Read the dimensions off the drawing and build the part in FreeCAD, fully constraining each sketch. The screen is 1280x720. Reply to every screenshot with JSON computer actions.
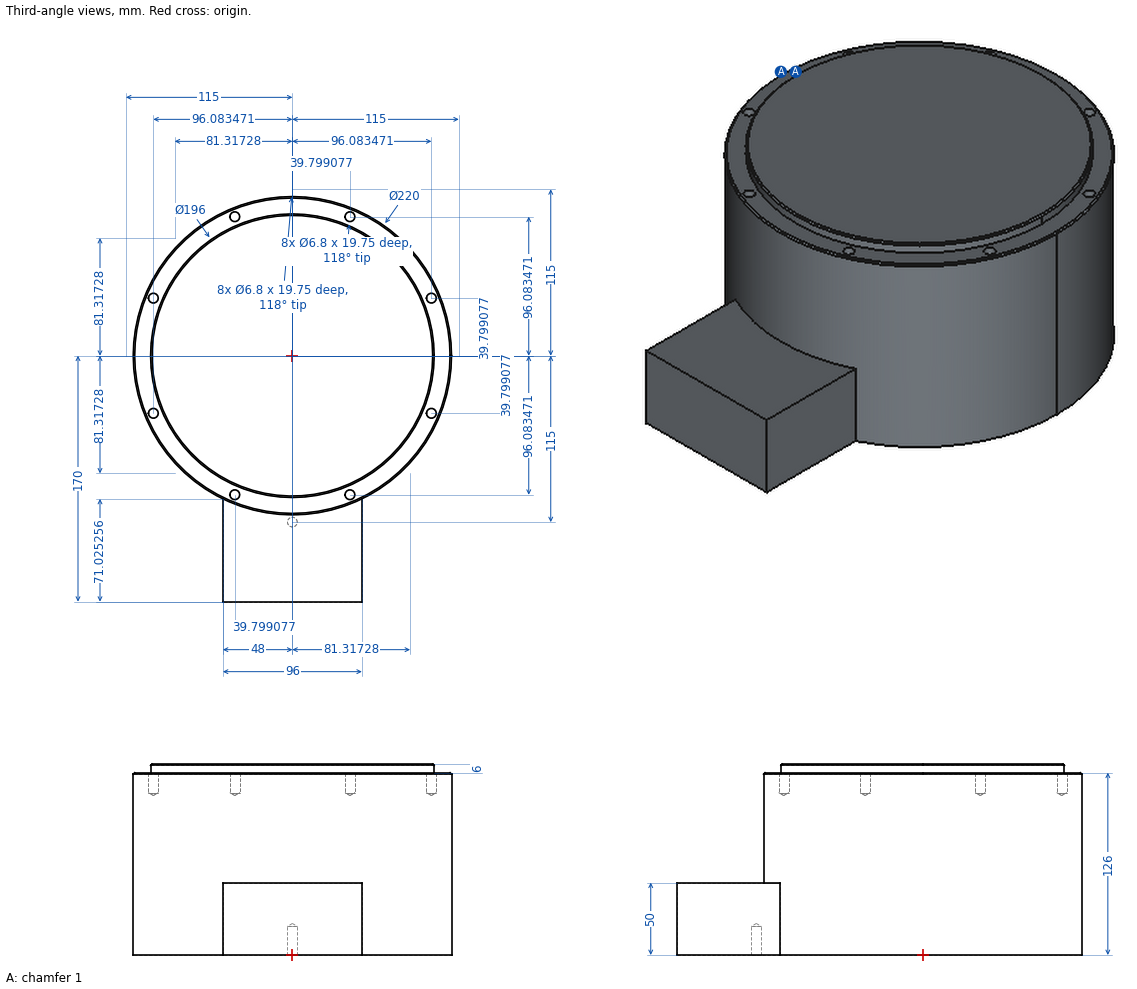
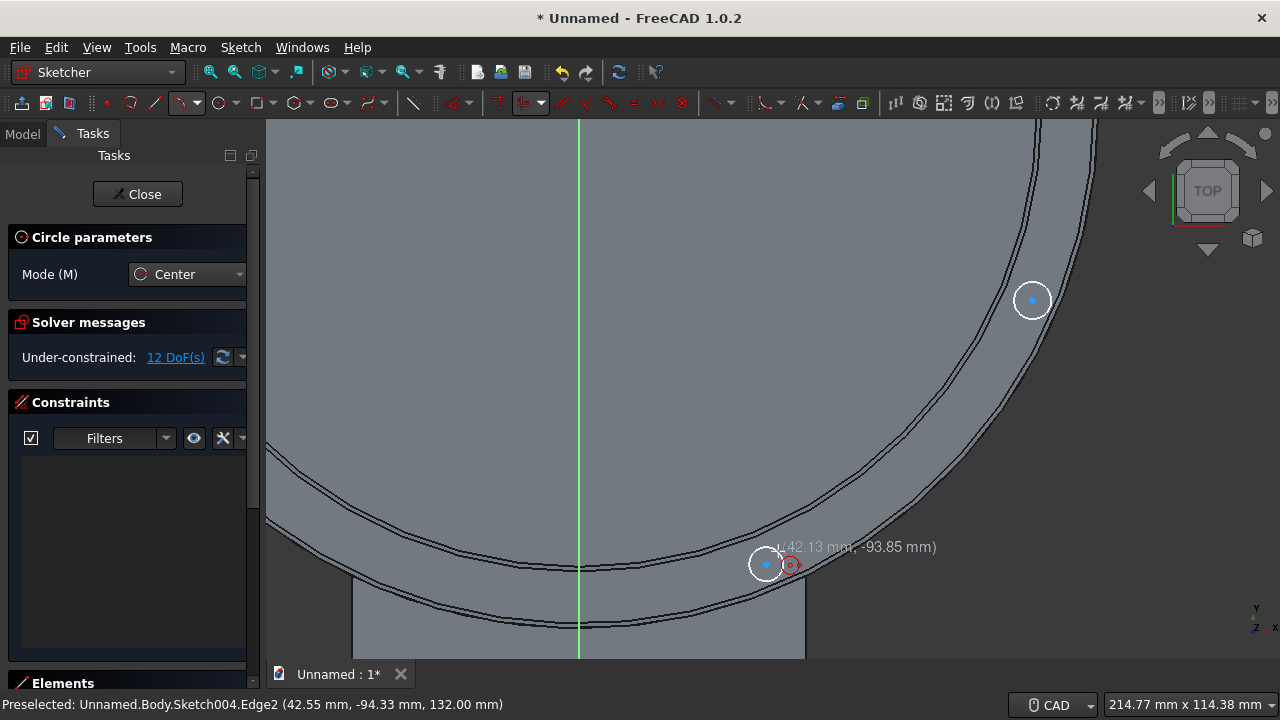
{"action": "scroll", "coordinate": [391, 563], "scroll_direction": "up", "scroll_amount": 2}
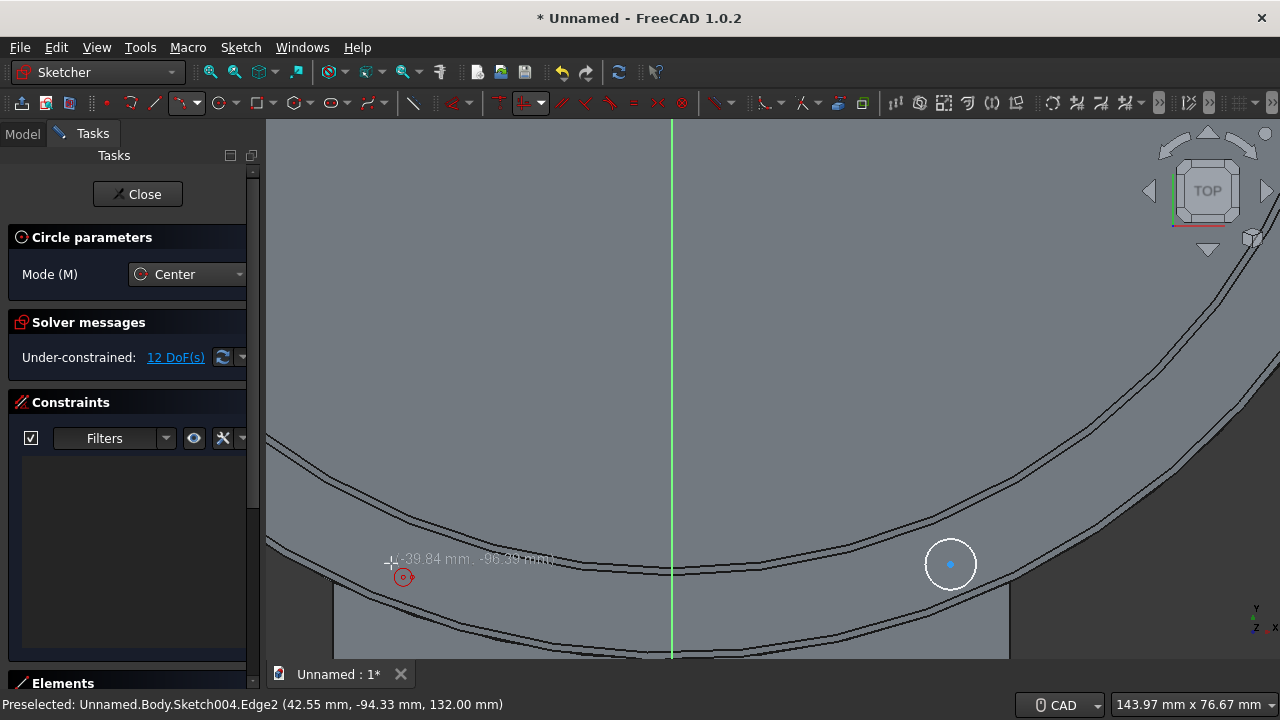
{"action": "scroll", "coordinate": [715, 554], "scroll_direction": "down", "scroll_amount": 7}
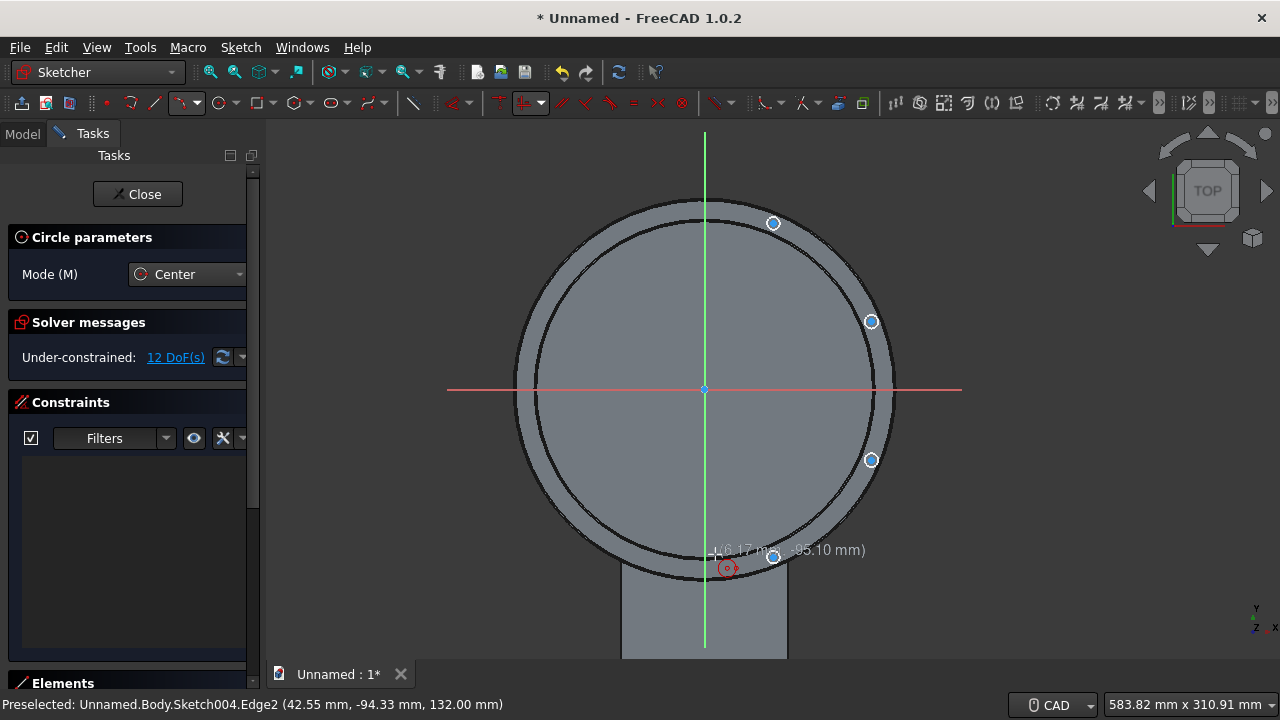
{"action": "left_click", "coordinate": [635, 557]}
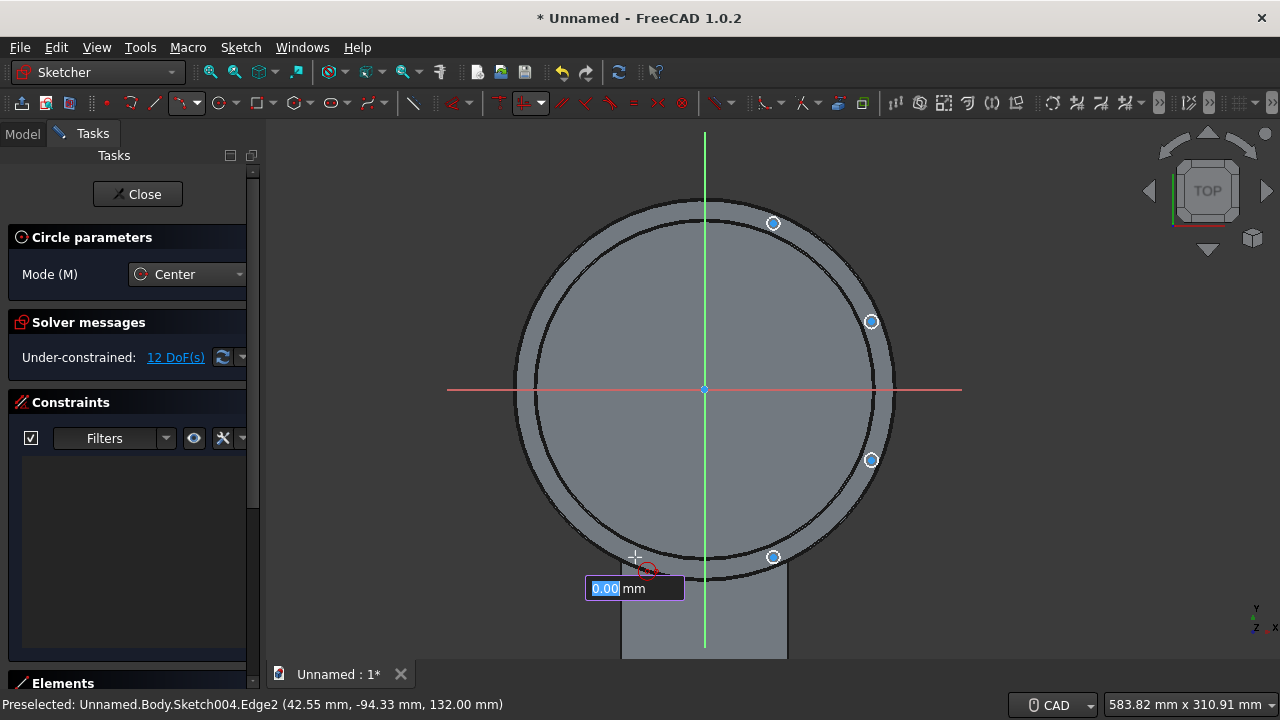
{"action": "scroll", "coordinate": [640, 552], "scroll_direction": "up", "scroll_amount": 5}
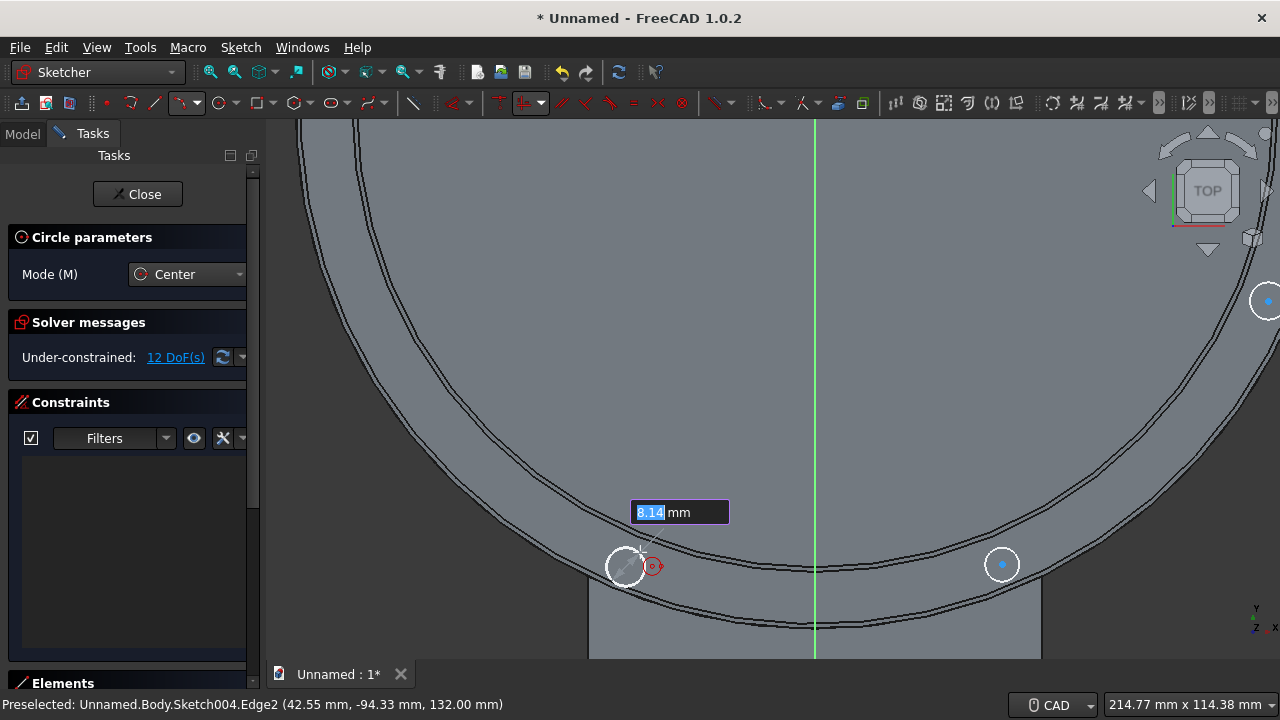
{"action": "left_click", "coordinate": [638, 552]}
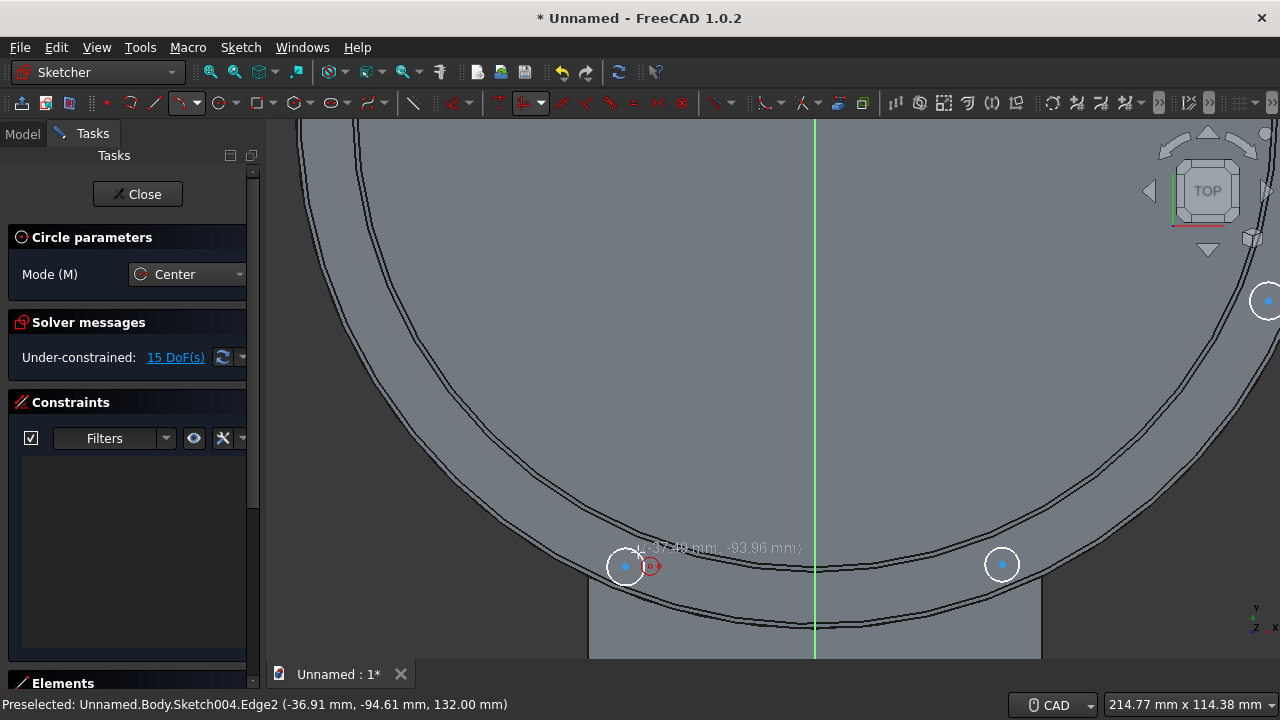
{"action": "scroll", "coordinate": [361, 297], "scroll_direction": "up", "scroll_amount": 2}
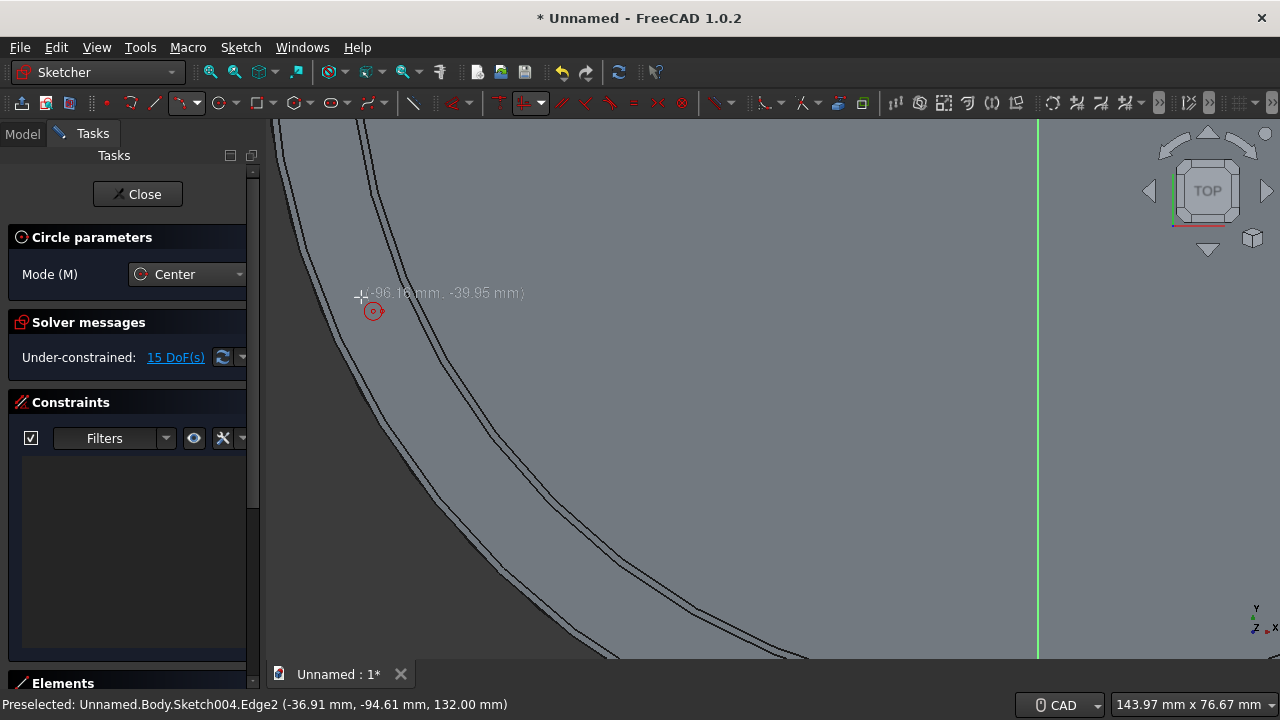
{"action": "scroll", "coordinate": [595, 511], "scroll_direction": "down", "scroll_amount": 7}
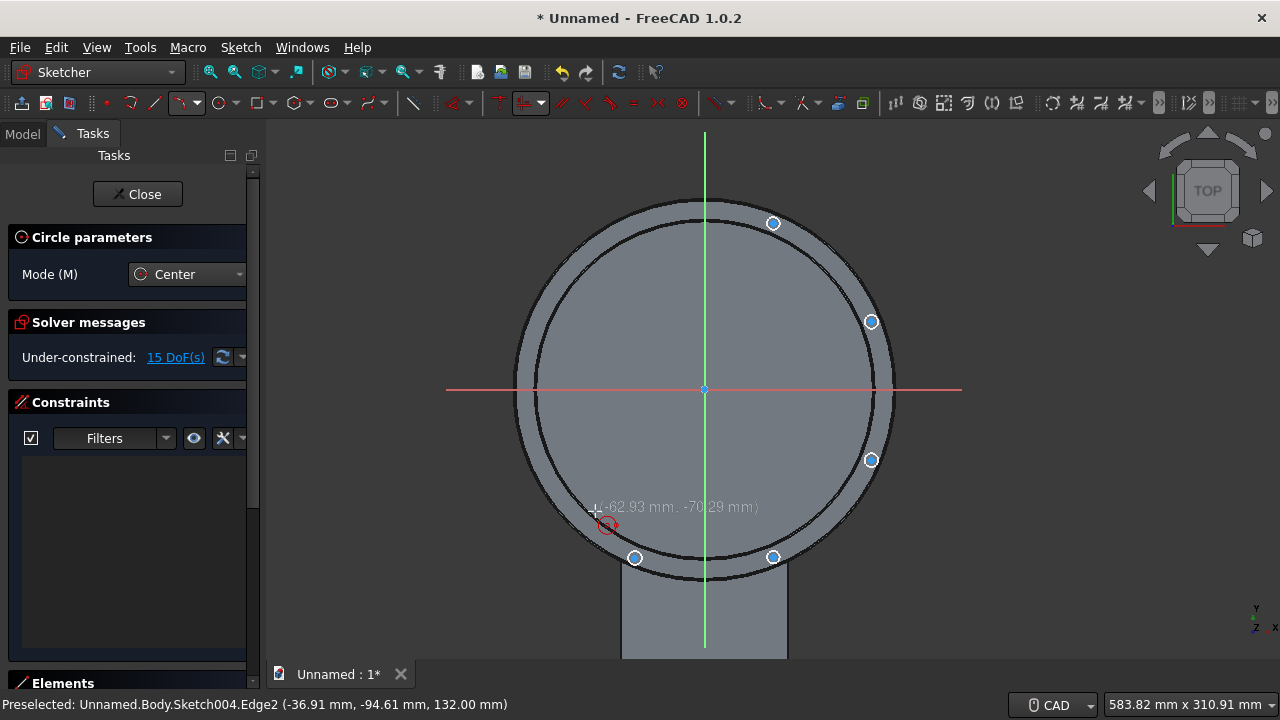
{"action": "left_click", "coordinate": [538, 459]}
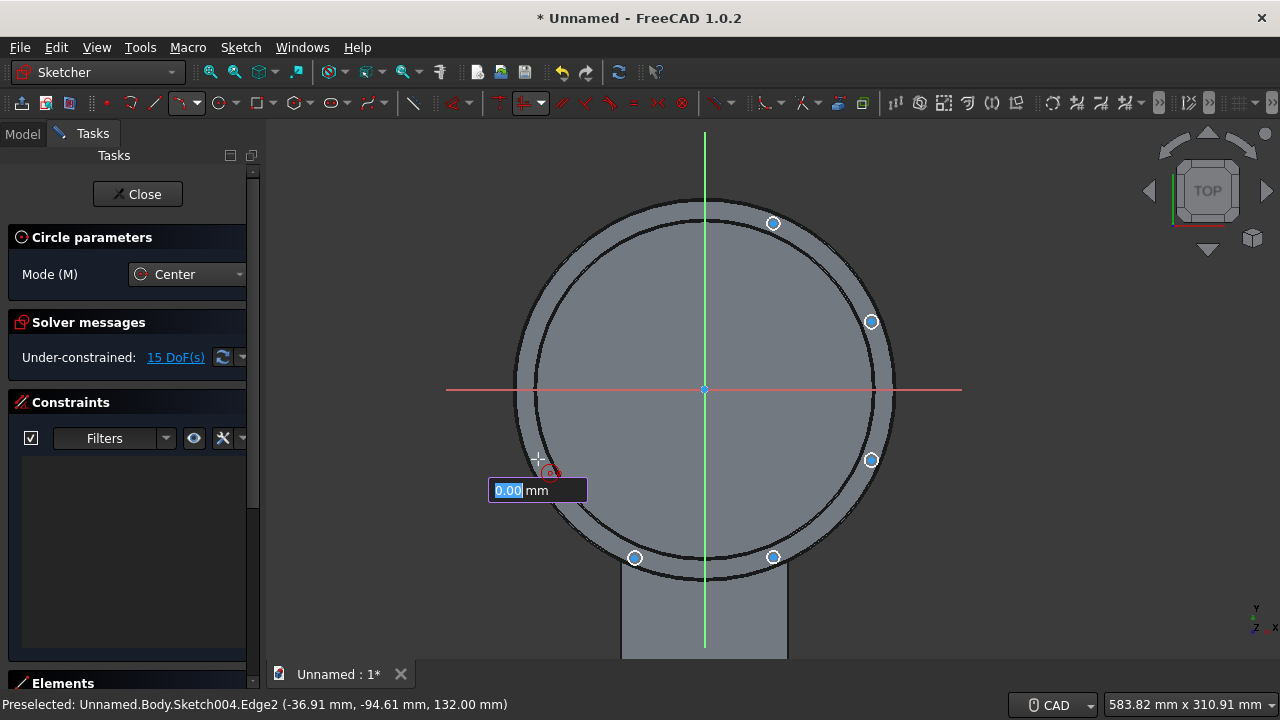
{"action": "scroll", "coordinate": [542, 455], "scroll_direction": "up", "scroll_amount": 5}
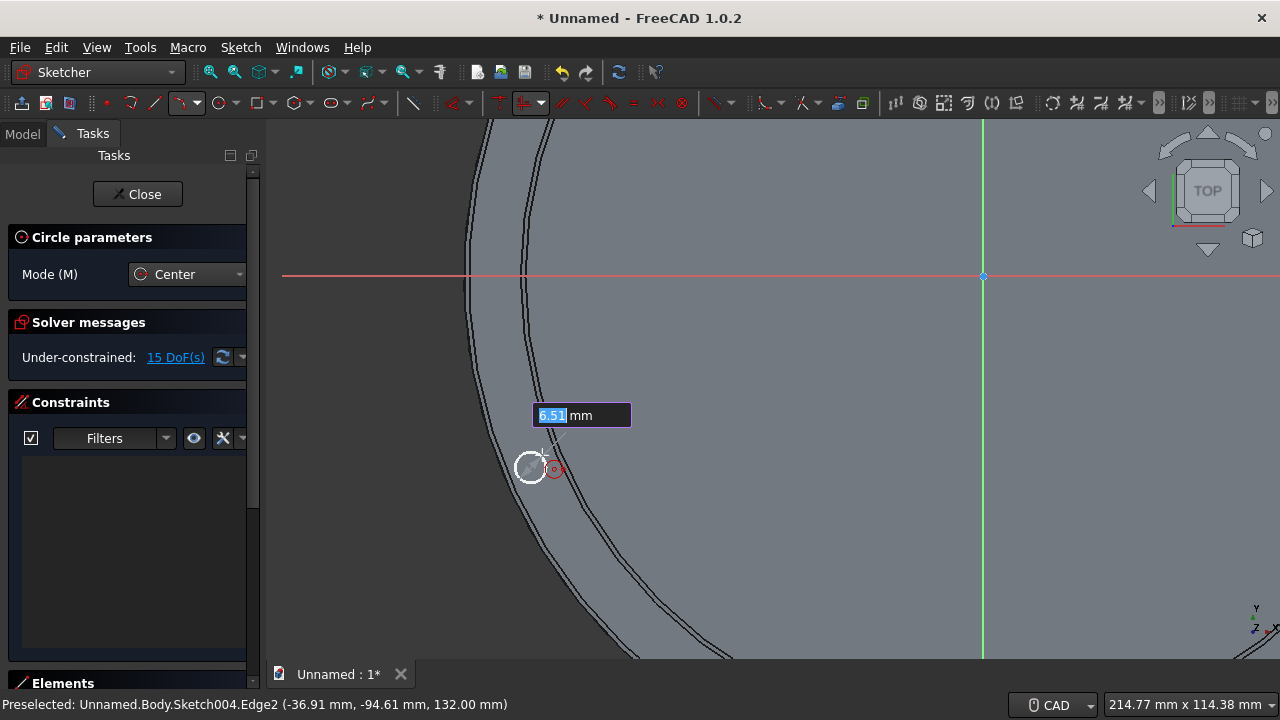
{"action": "left_click", "coordinate": [541, 453]}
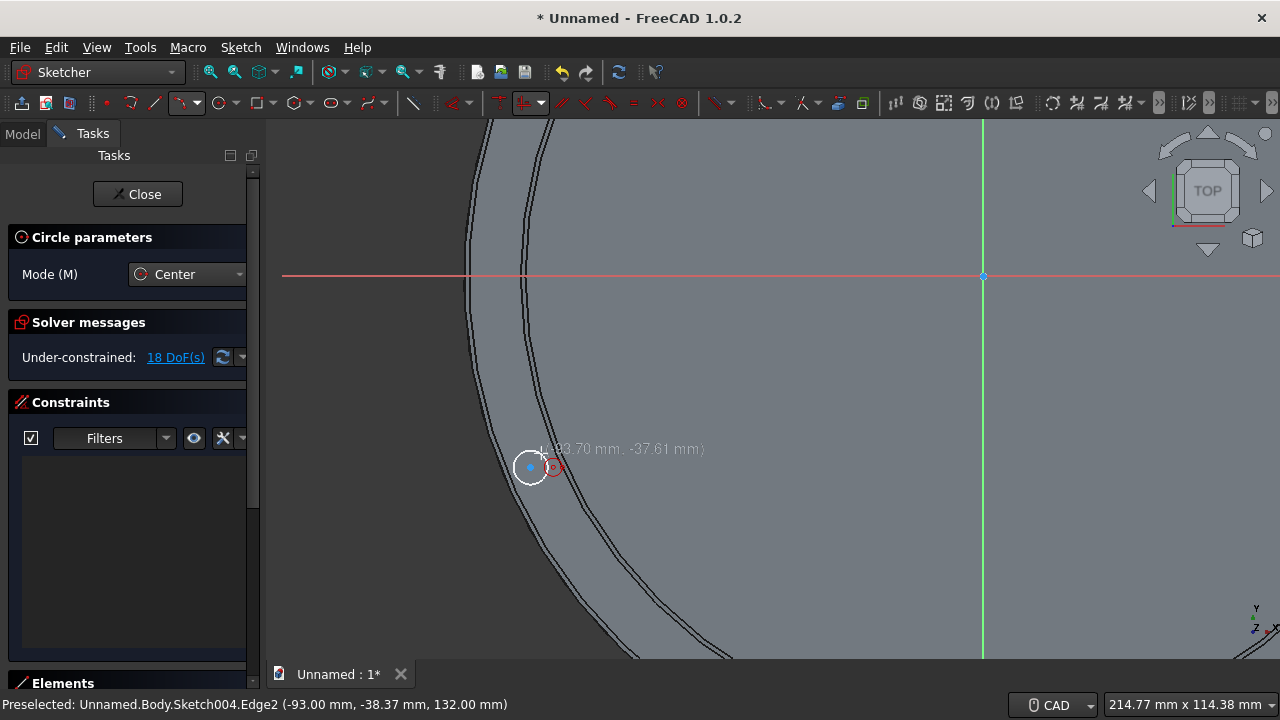
{"action": "scroll", "coordinate": [542, 454], "scroll_direction": "down", "scroll_amount": 5}